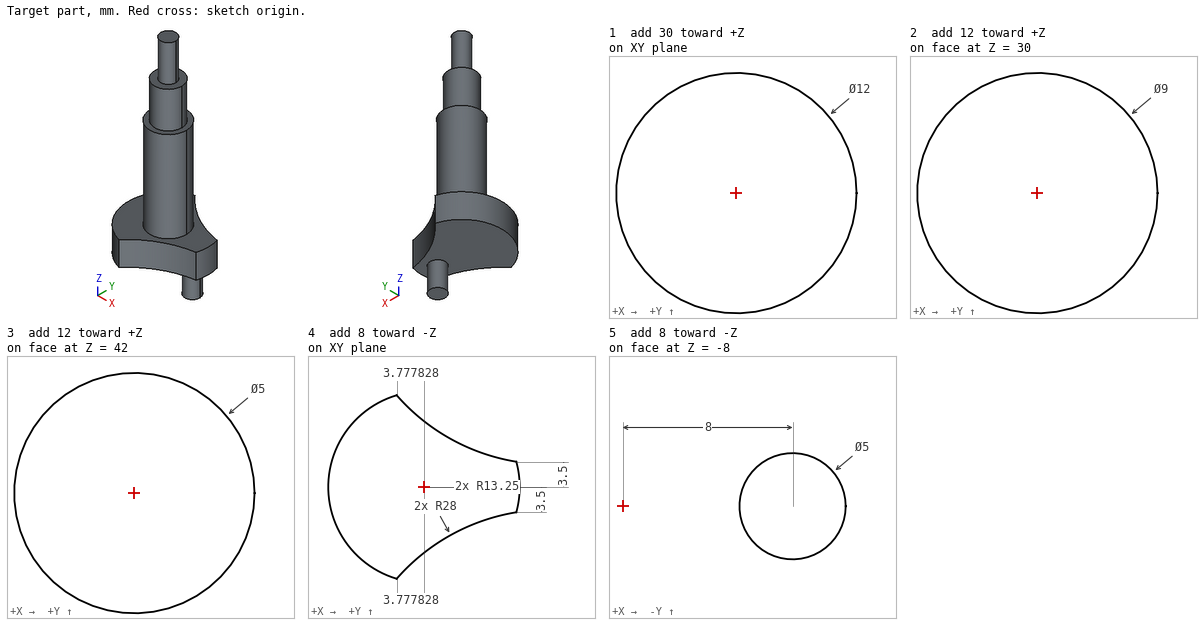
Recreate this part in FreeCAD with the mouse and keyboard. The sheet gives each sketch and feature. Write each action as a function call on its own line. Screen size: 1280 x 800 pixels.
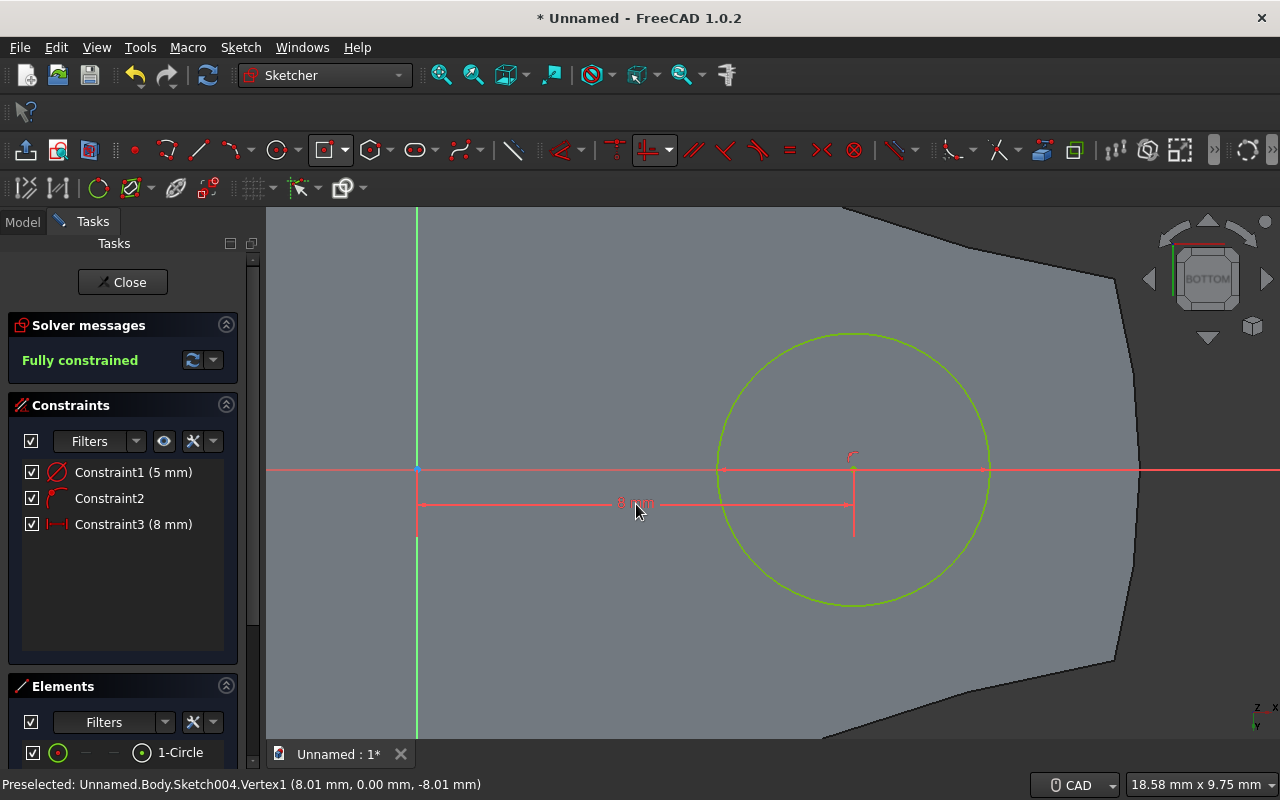
click(123, 282)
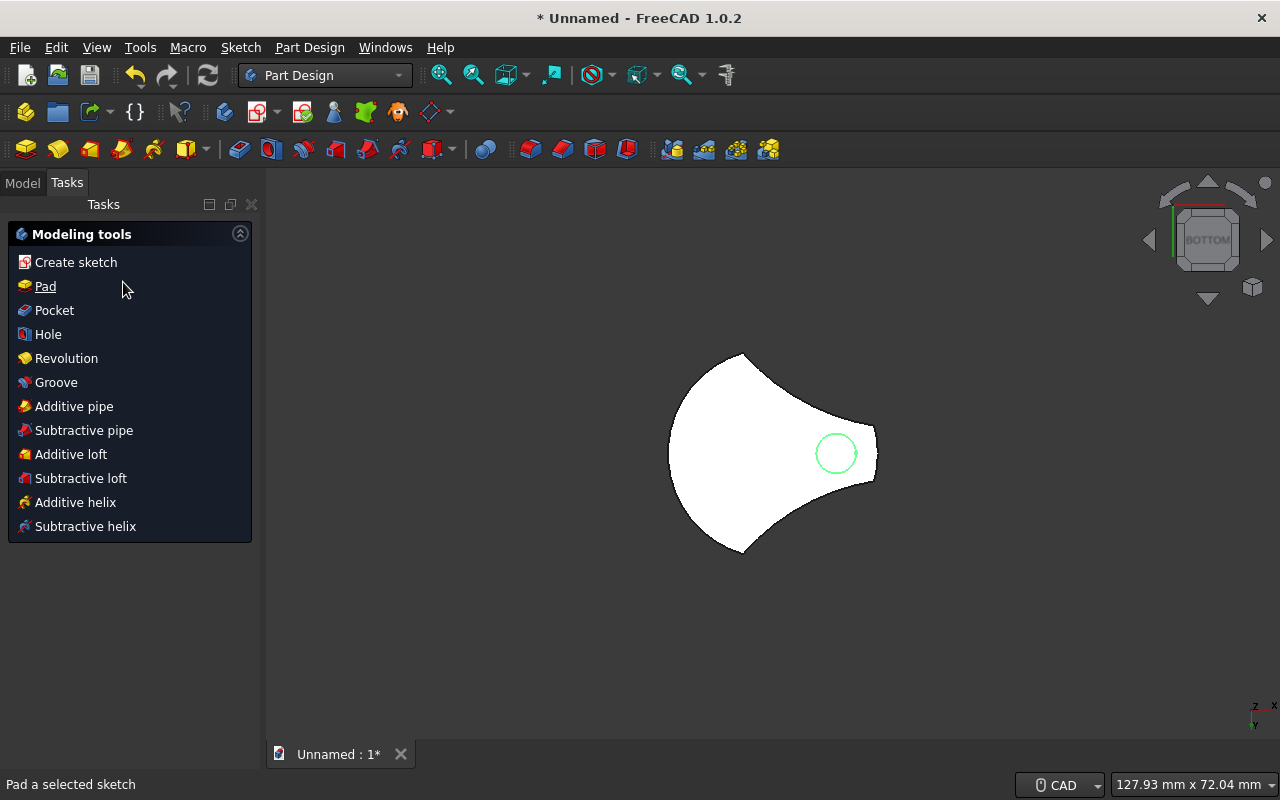
click(26, 150)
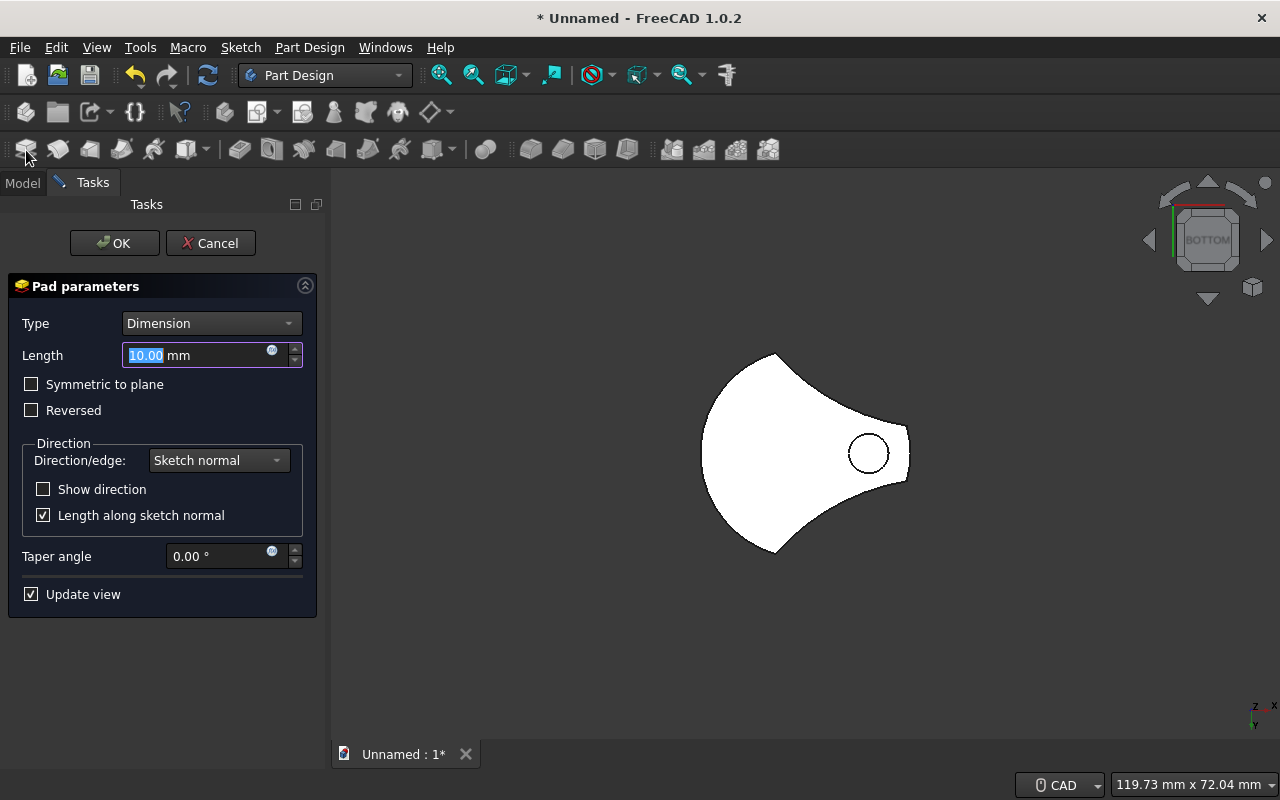
text(8)
key(Tab)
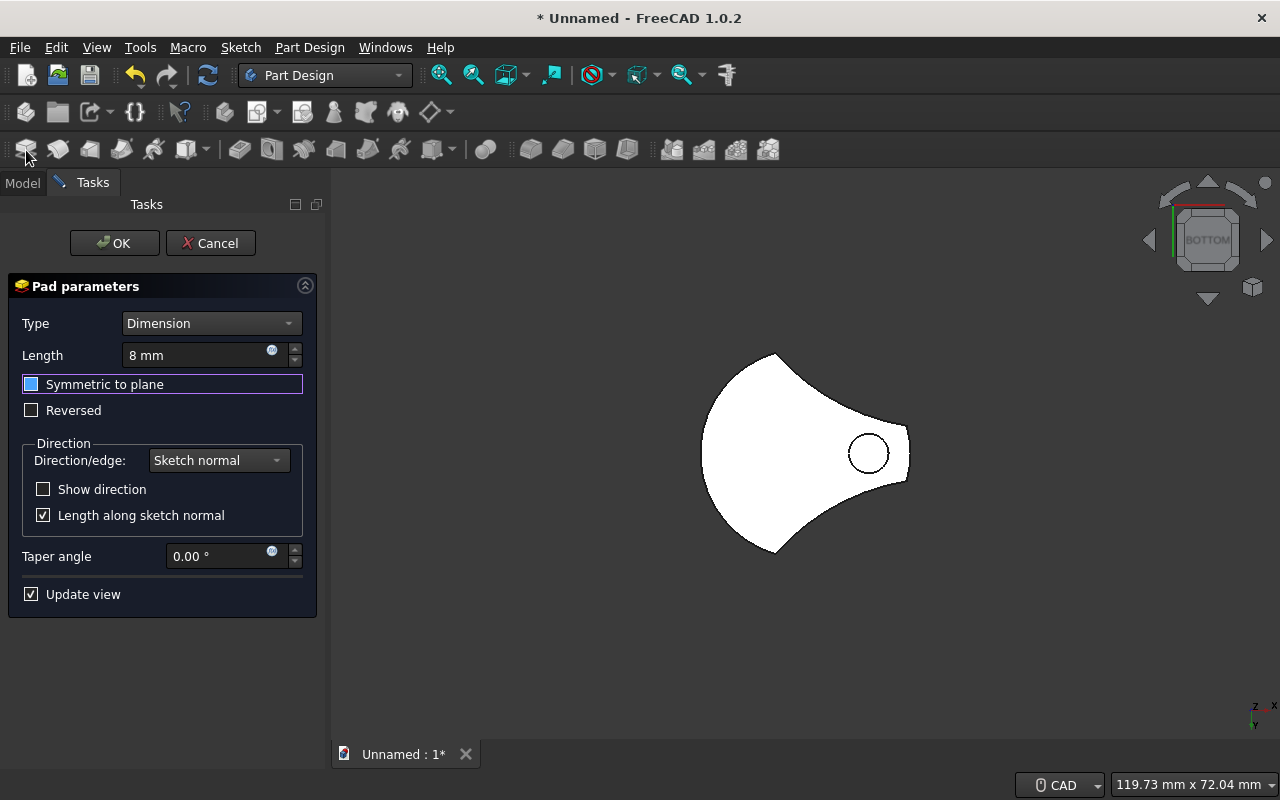
click(115, 243)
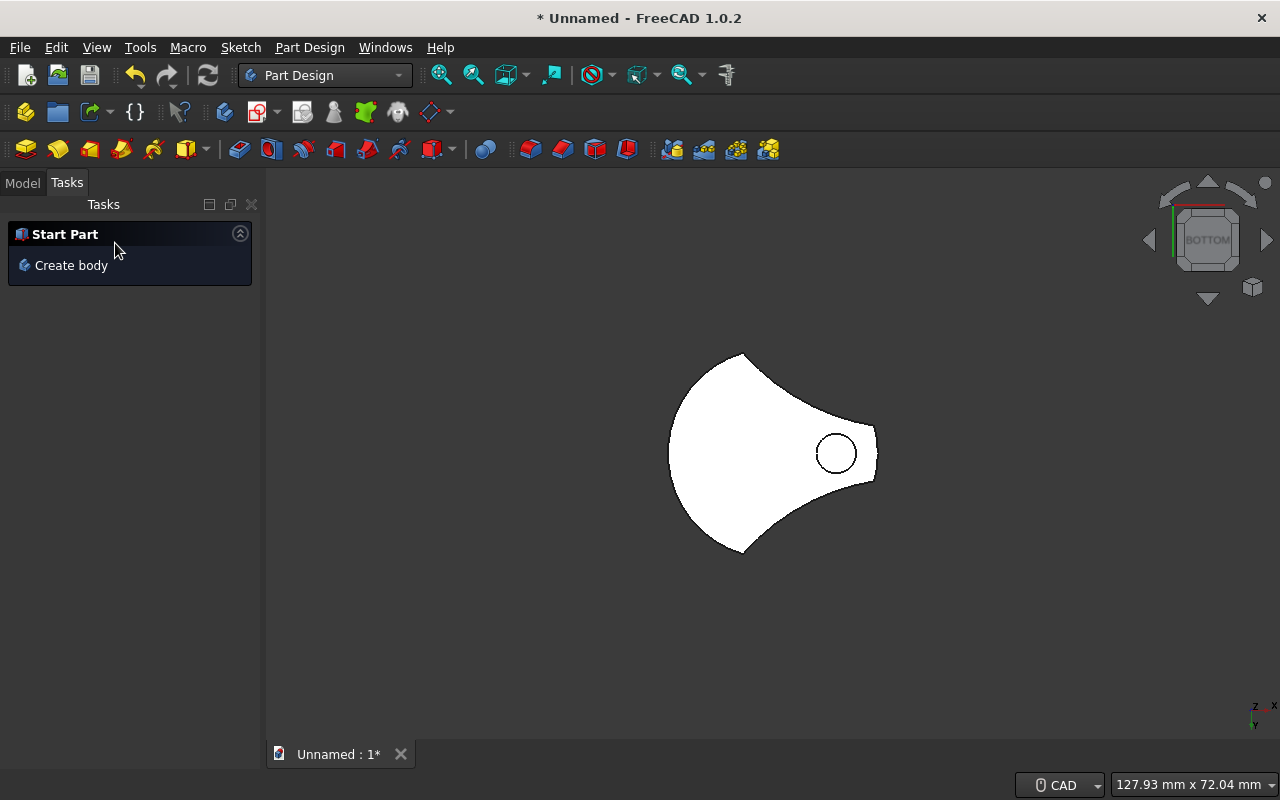
key(0)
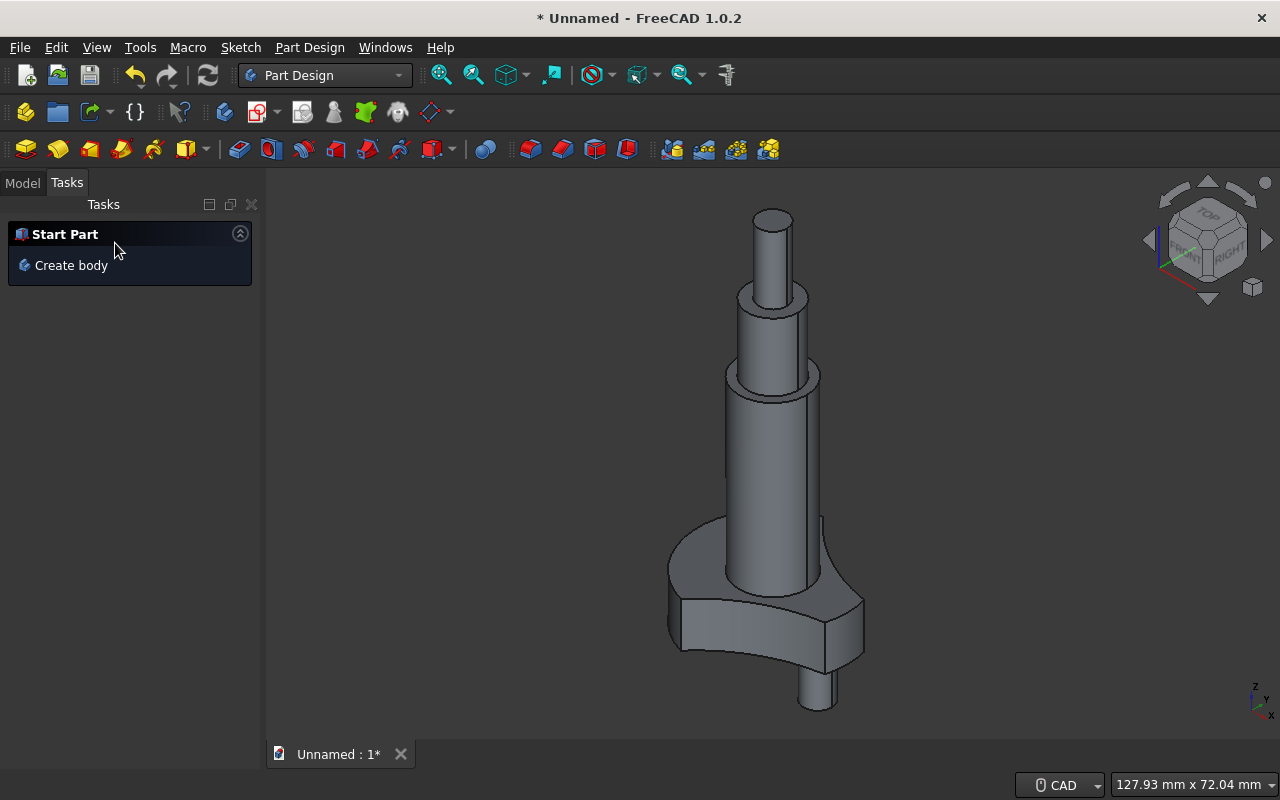
click(442, 76)